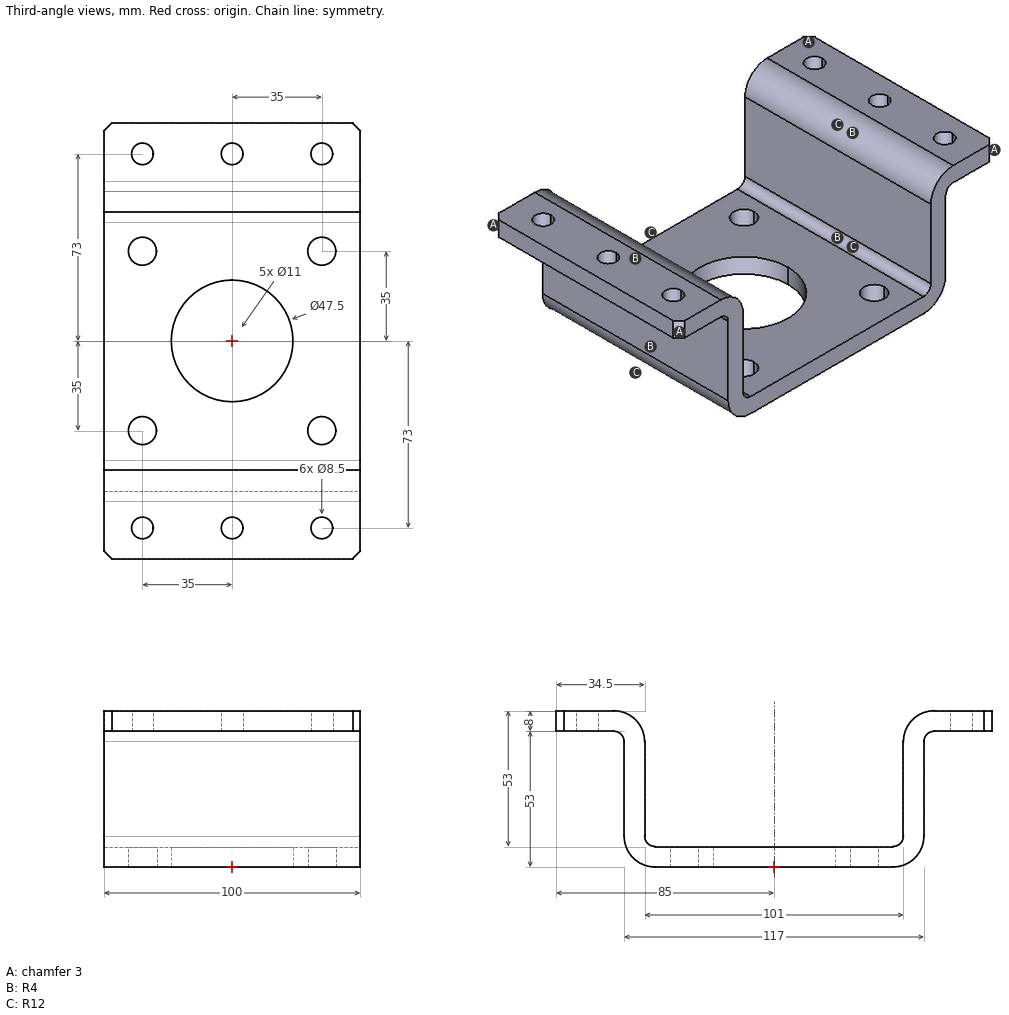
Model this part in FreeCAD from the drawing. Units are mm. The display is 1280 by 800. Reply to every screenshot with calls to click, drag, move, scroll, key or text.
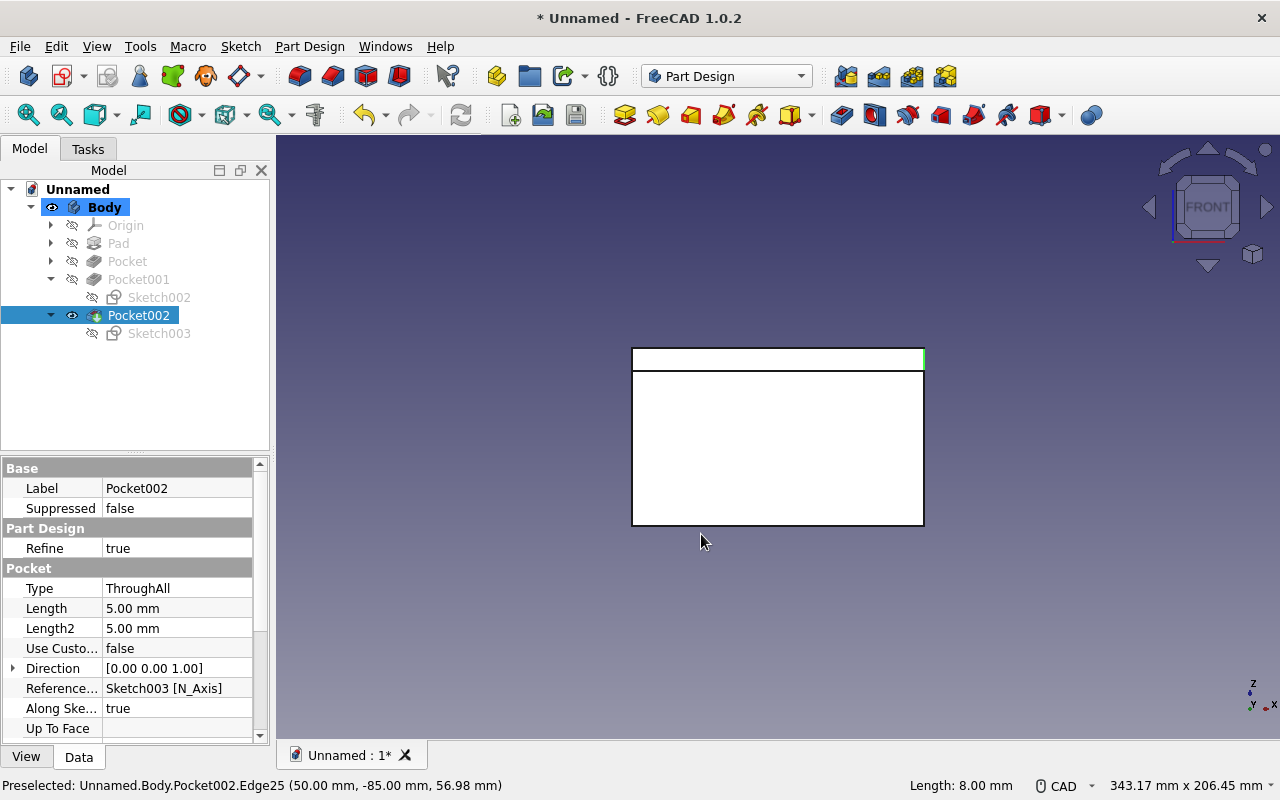
key(v)
key(f)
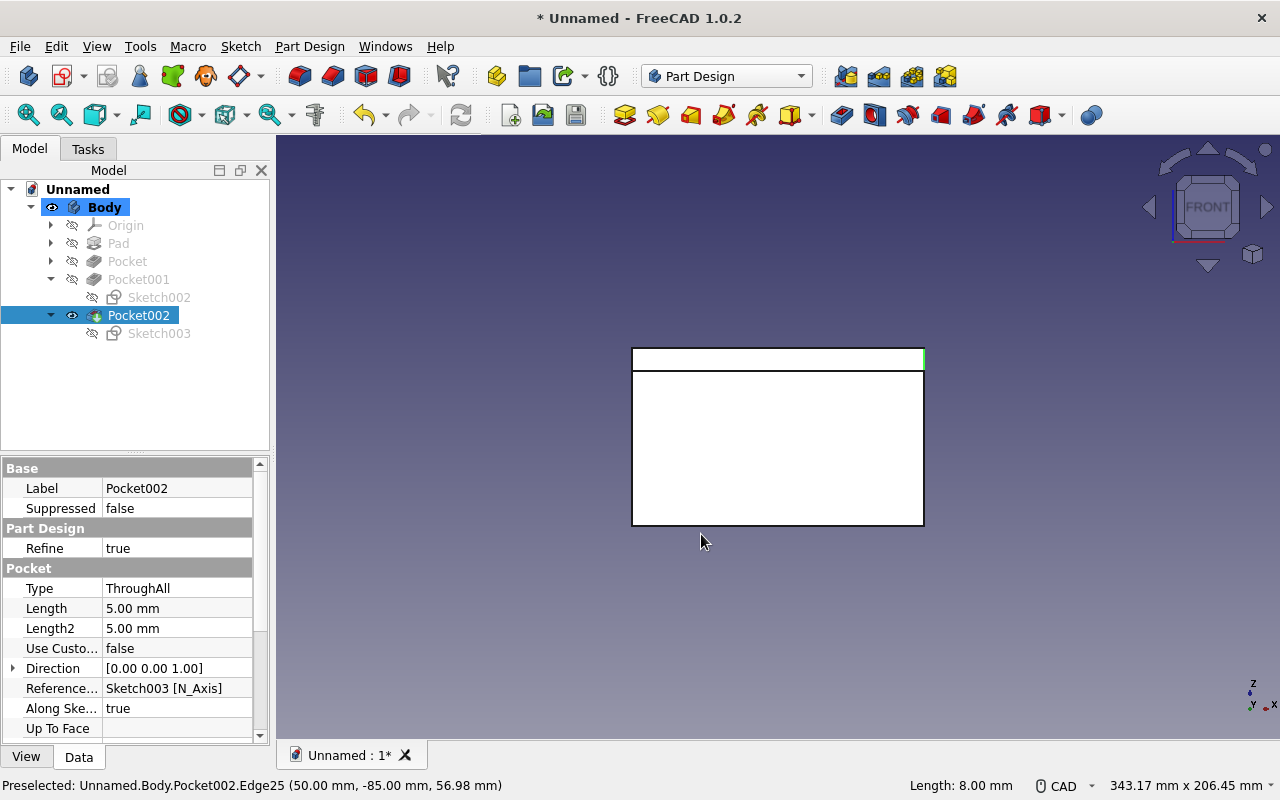
click(632, 358, ctrl)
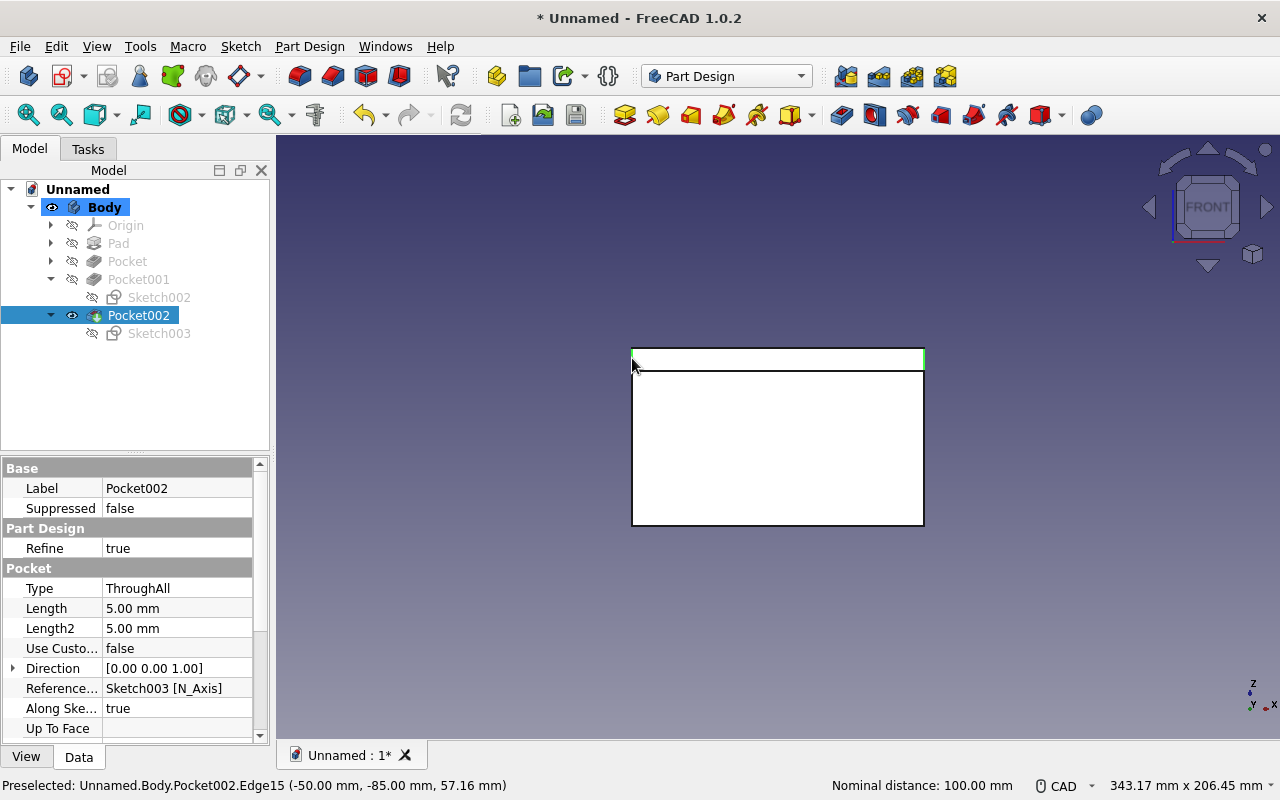
key(3)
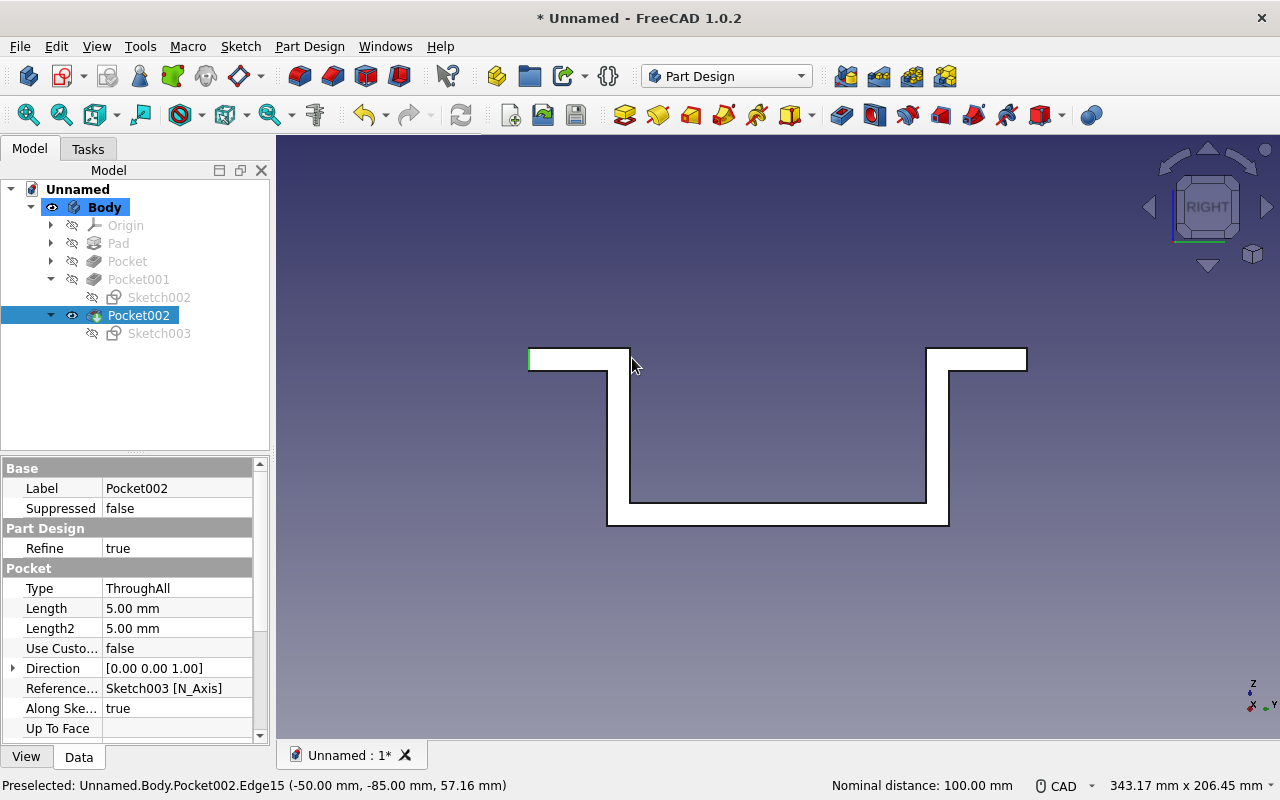
click(1027, 358, ctrl)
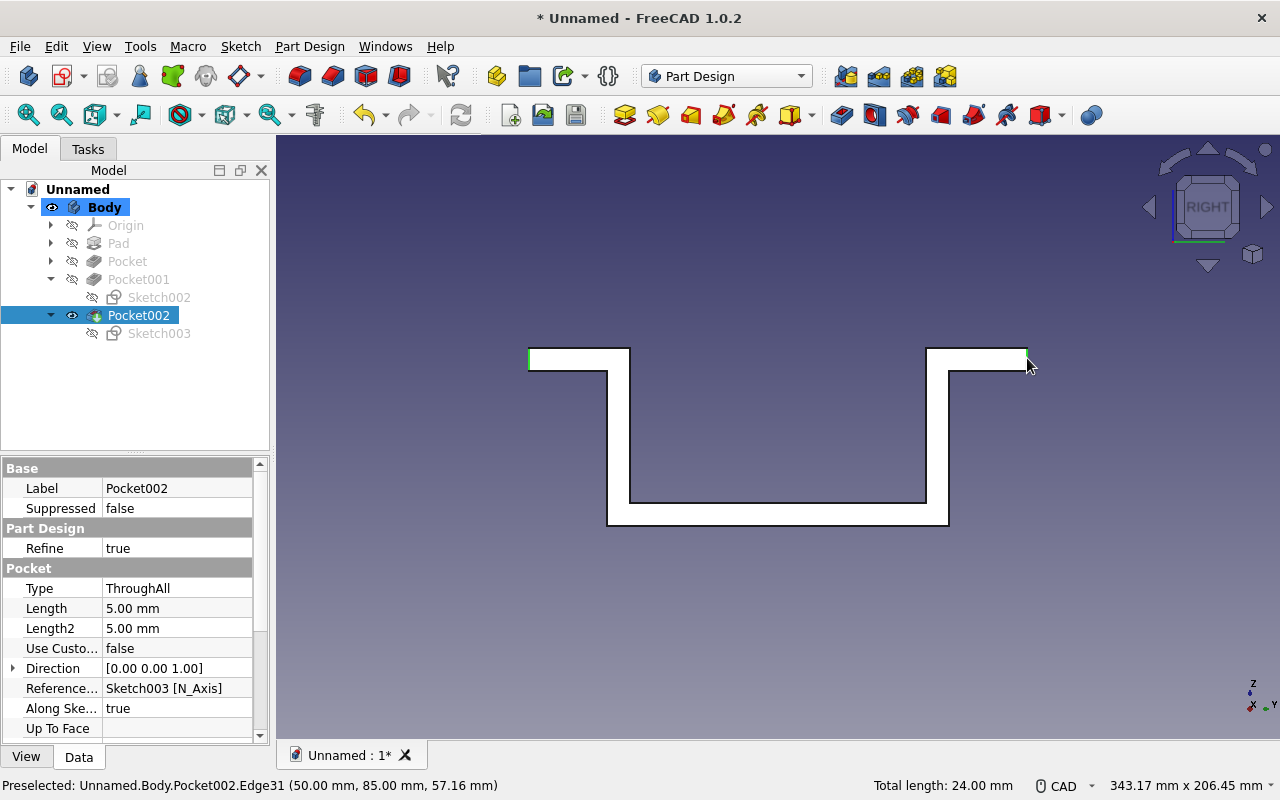
key(5)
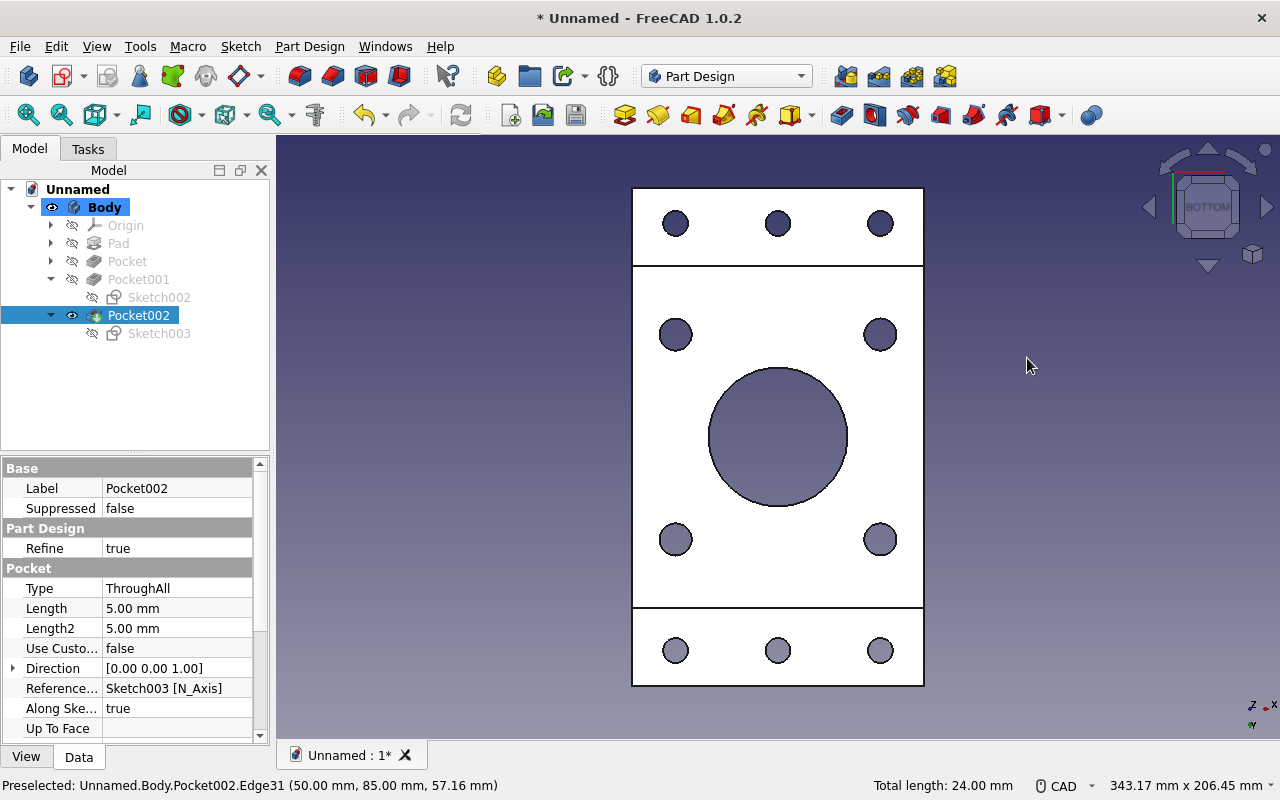
key(4)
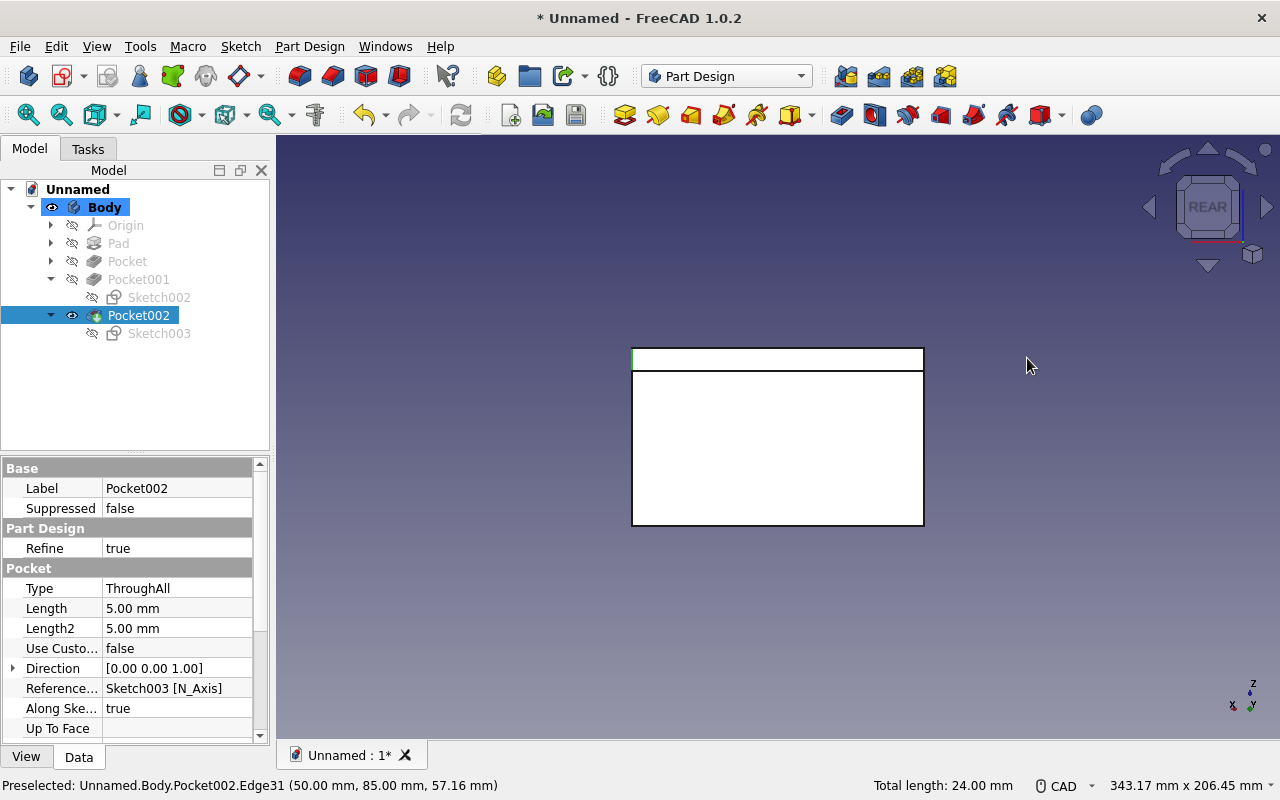
click(29, 116)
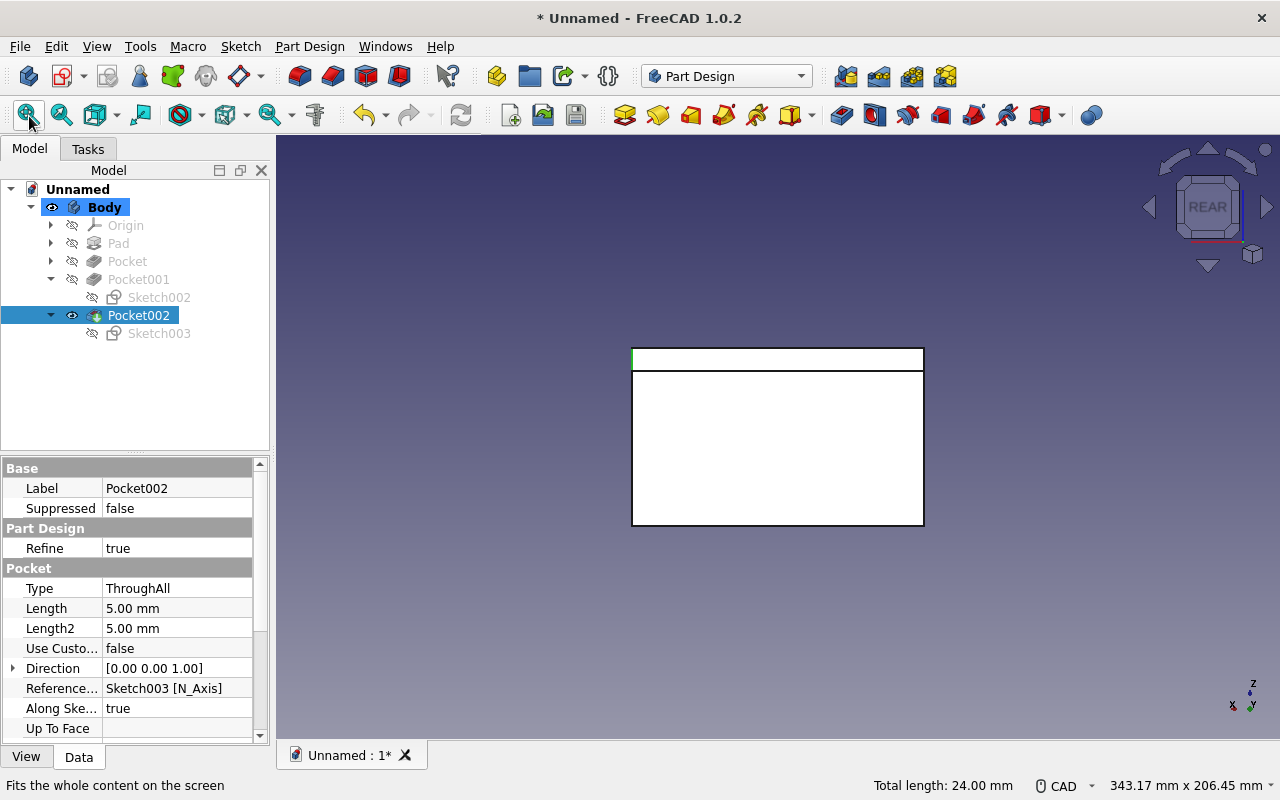
click(924, 358, ctrl)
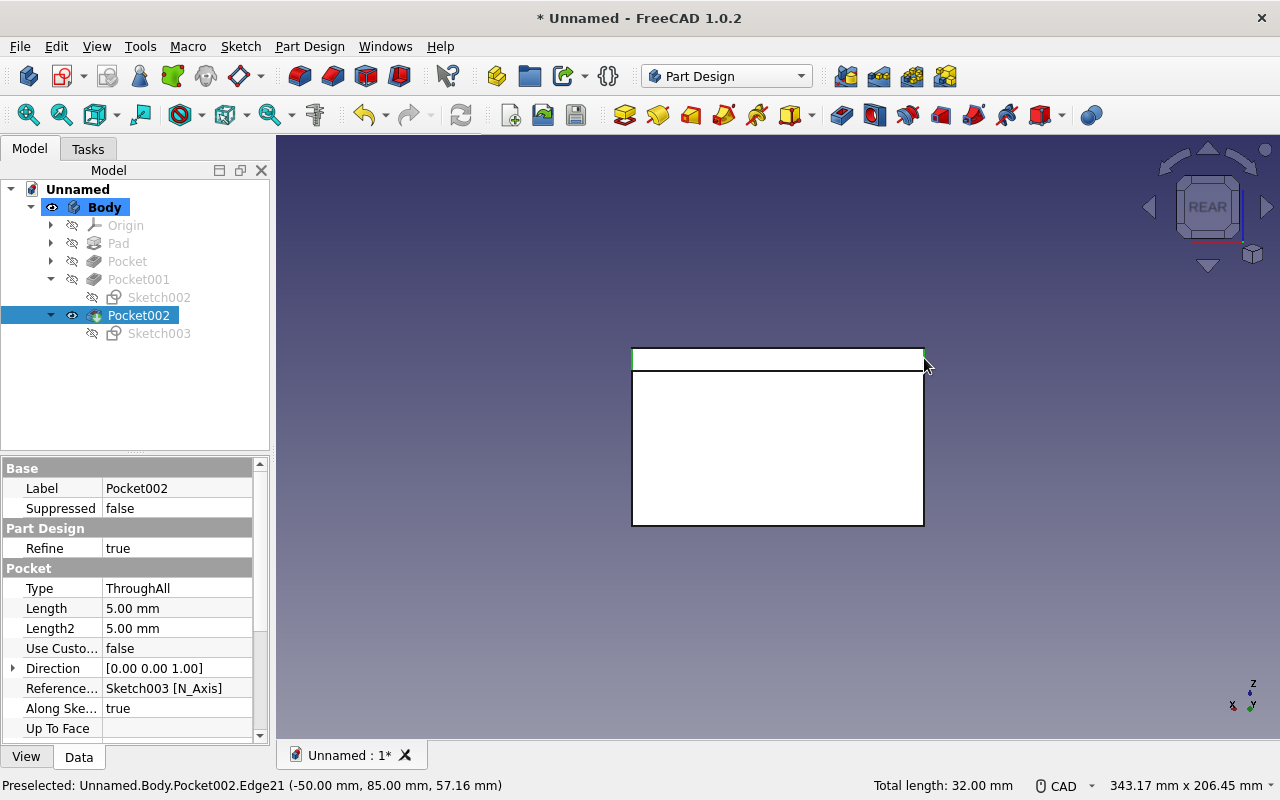
click(333, 76)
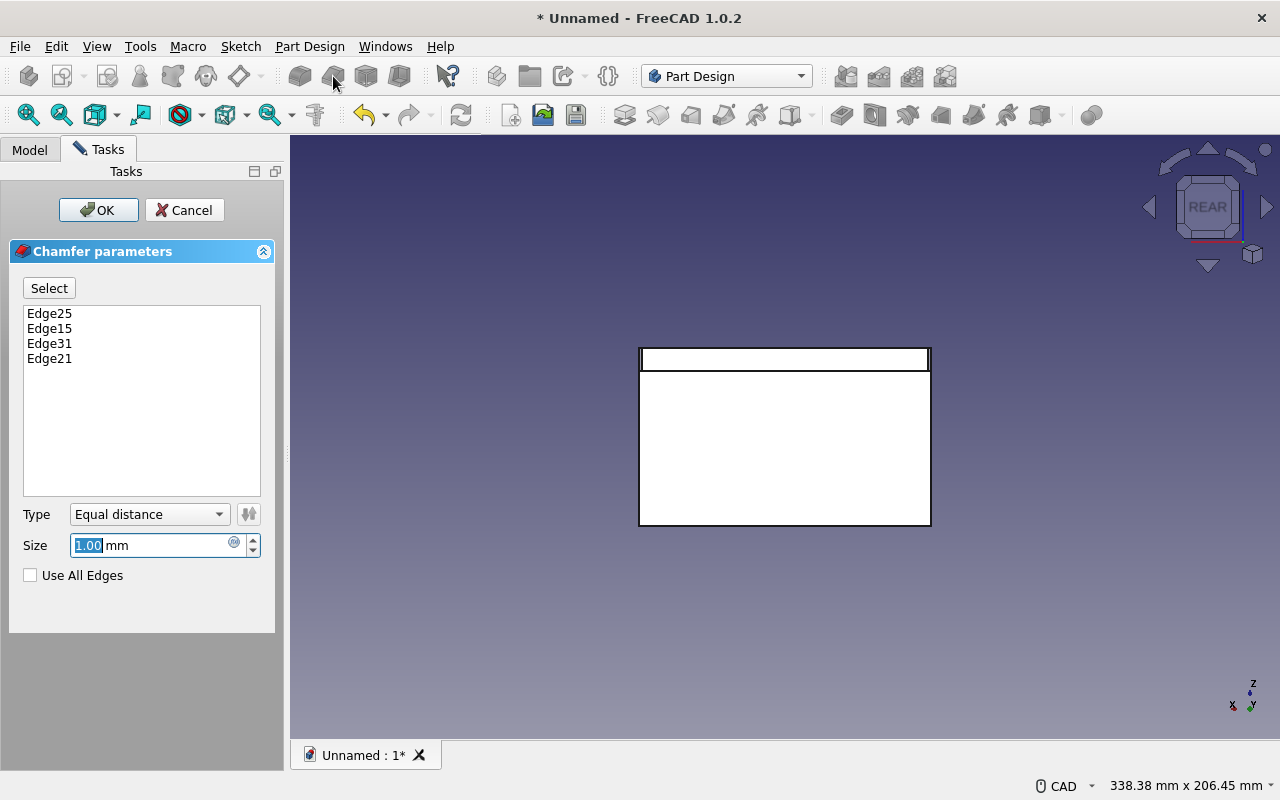
text(3)
key(Tab)